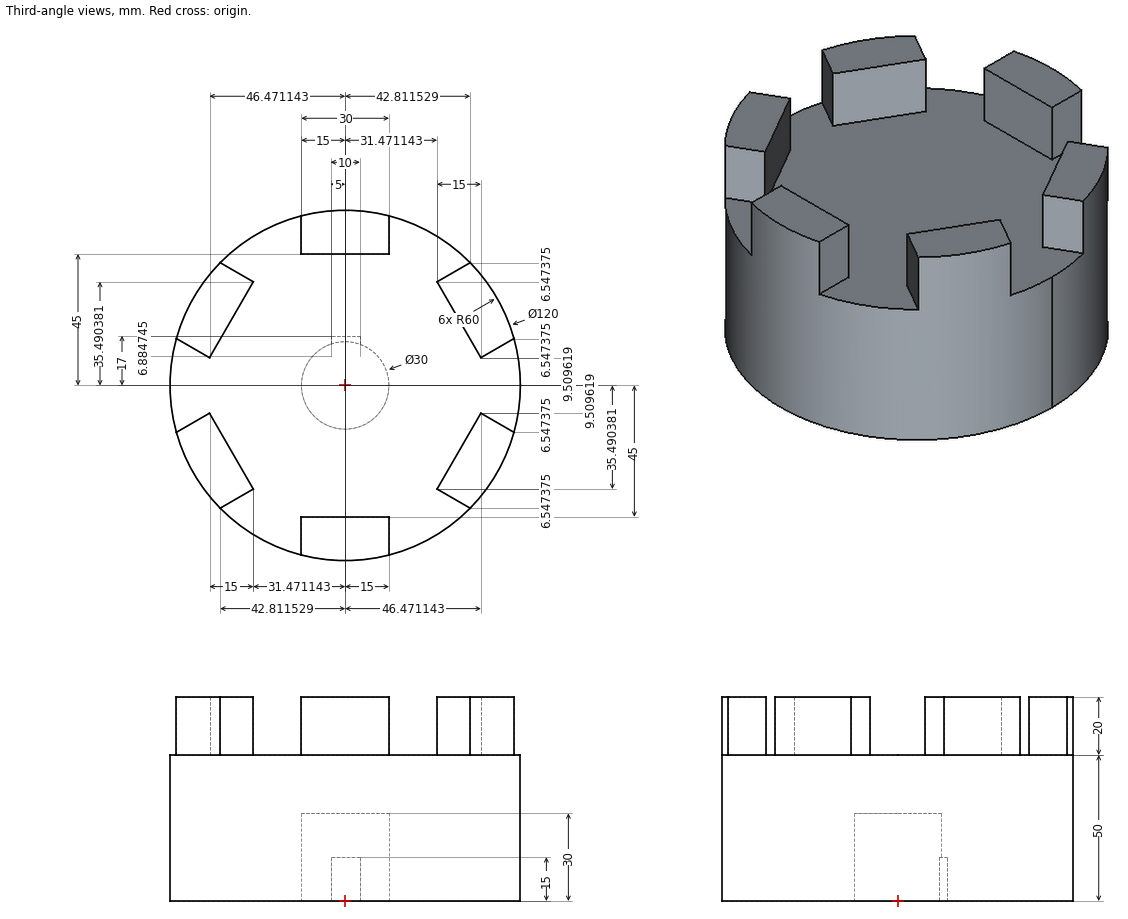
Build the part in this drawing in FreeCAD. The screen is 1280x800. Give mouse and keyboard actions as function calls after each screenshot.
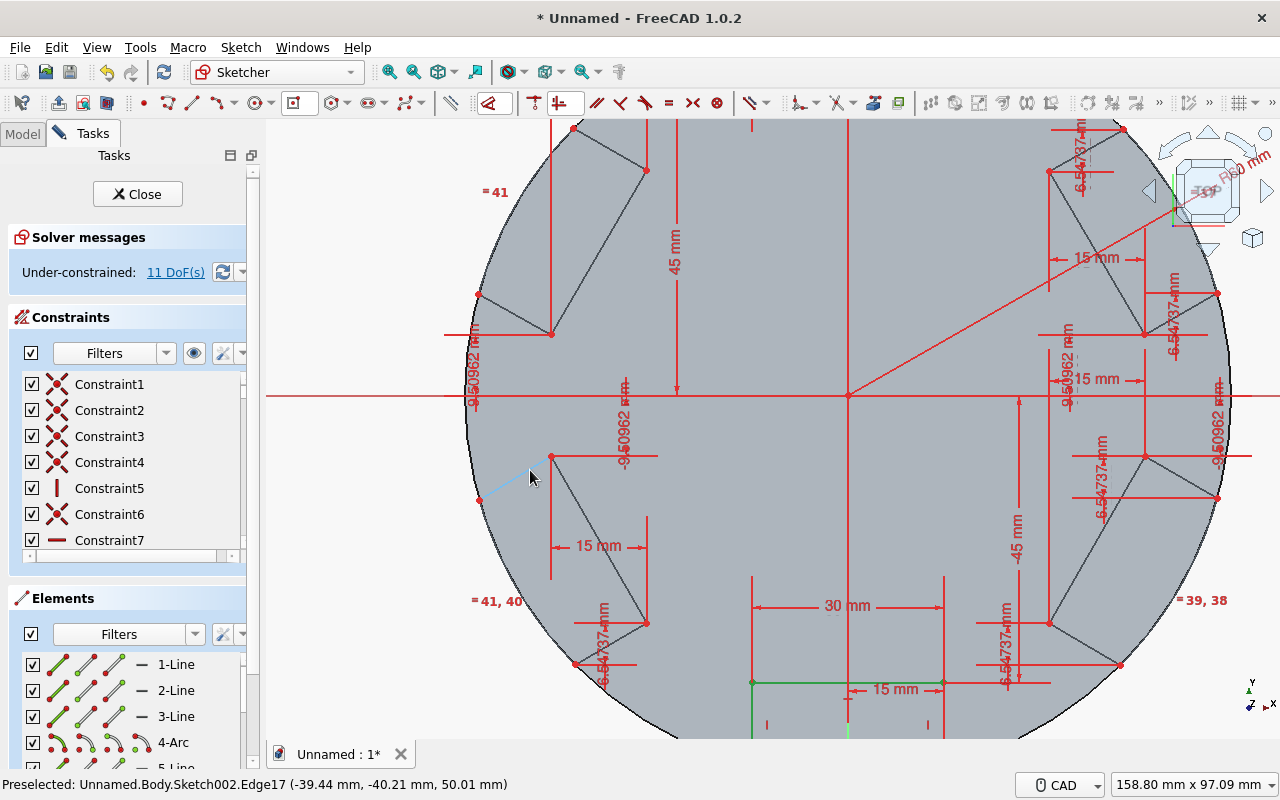
click(530, 470)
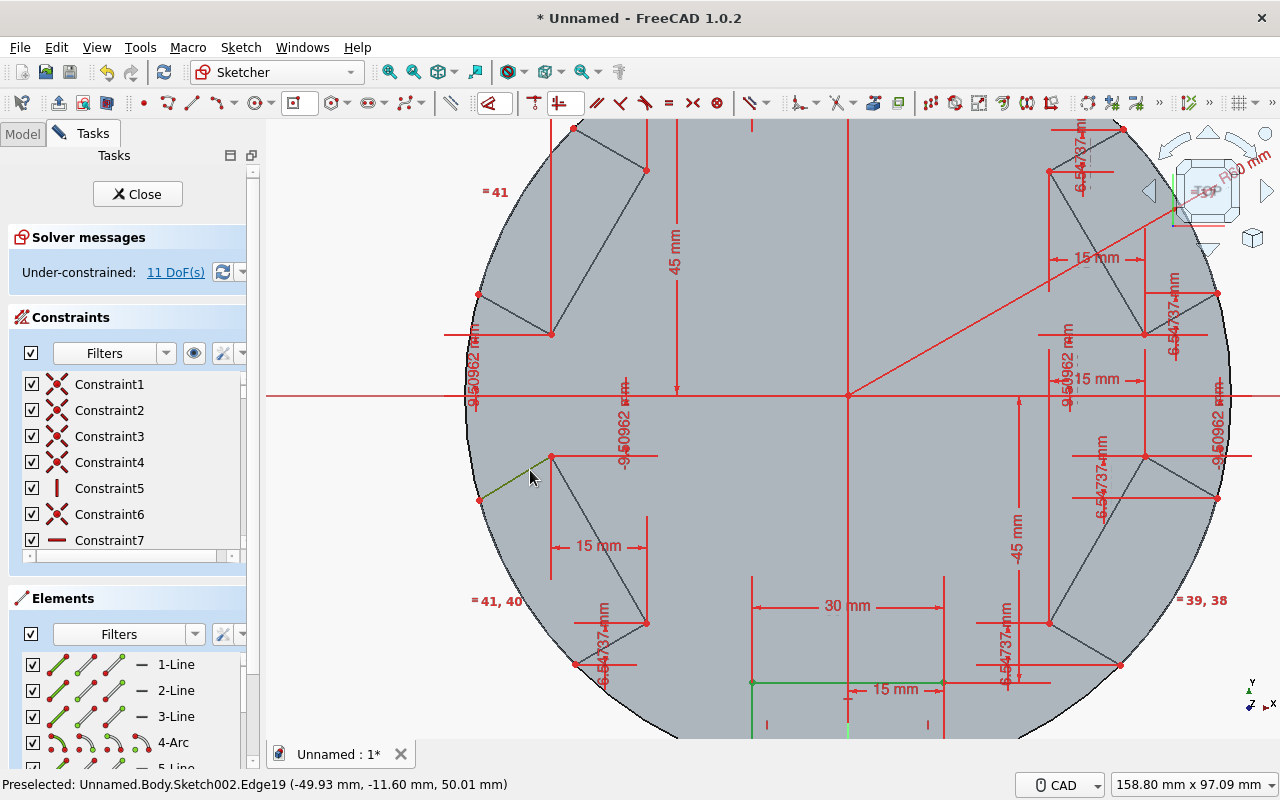
key(i)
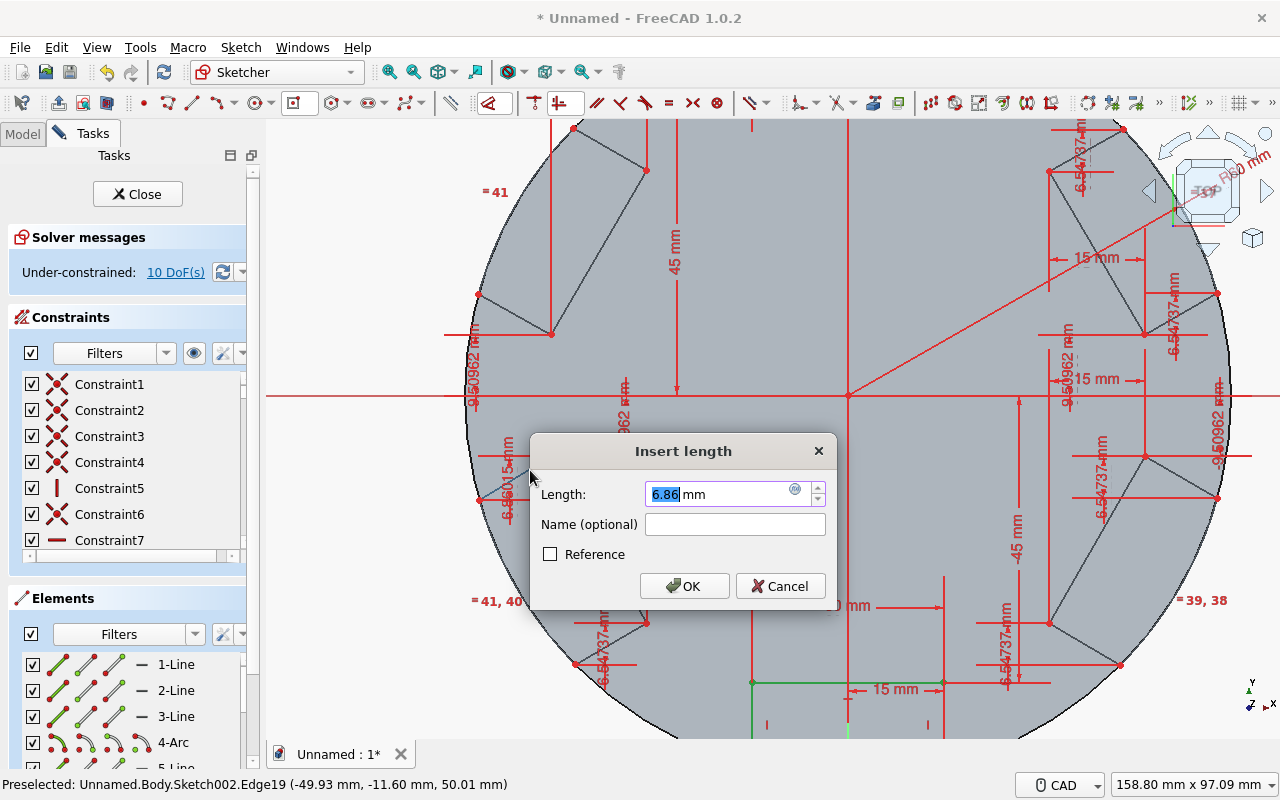
text(6.547375)
key(Return)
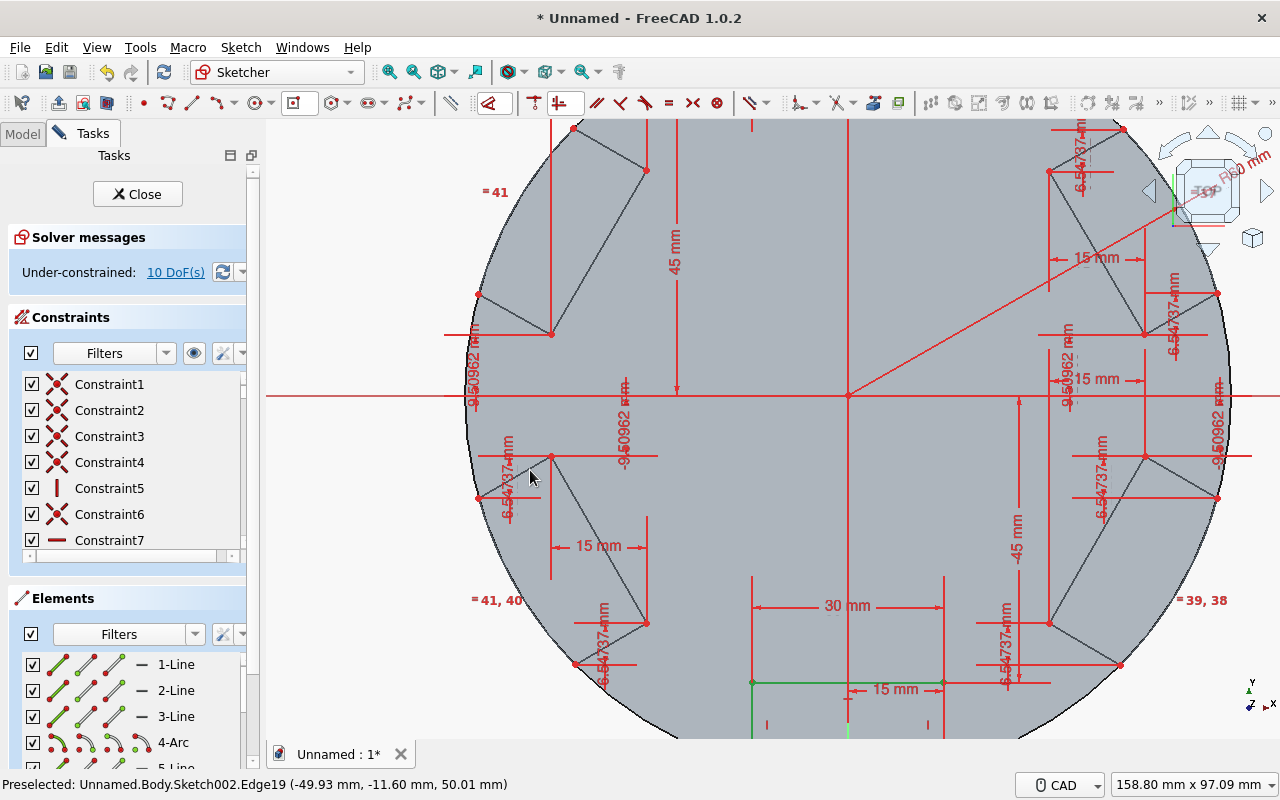
click(500, 306)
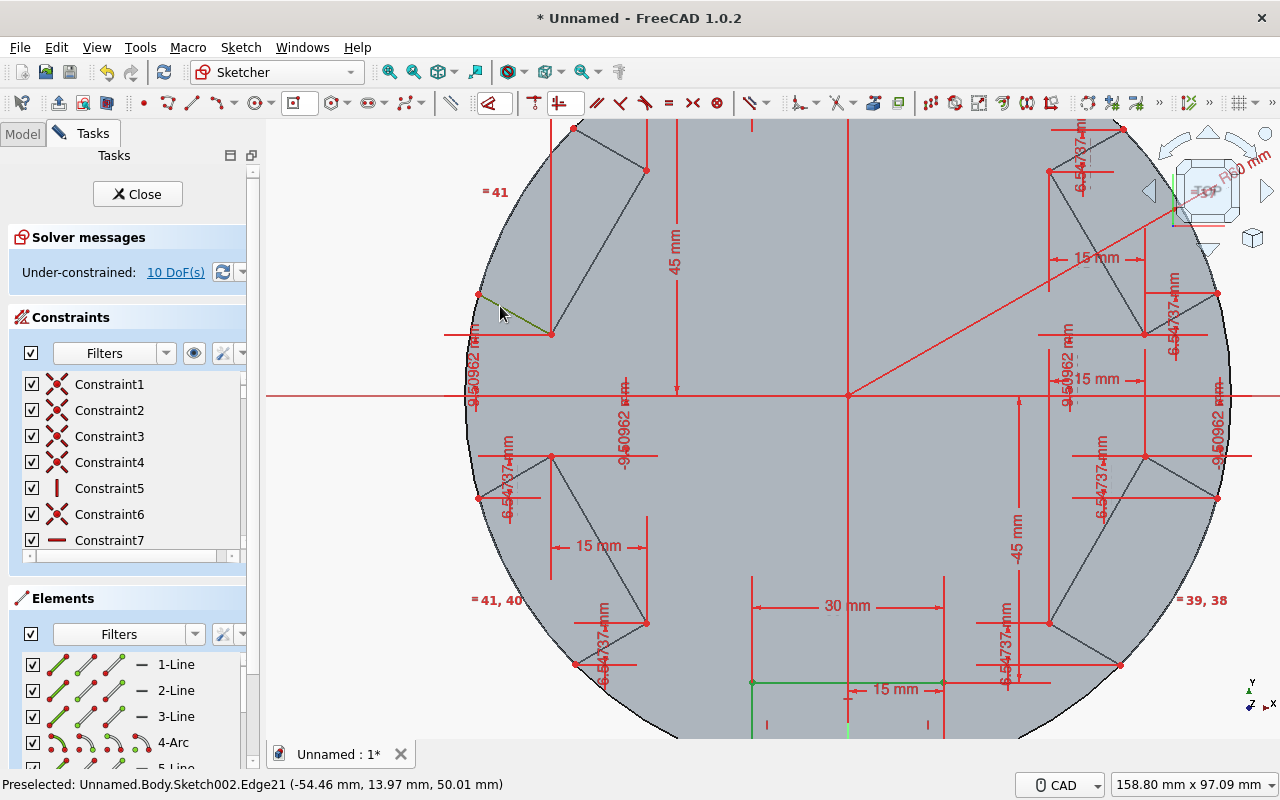
key(i)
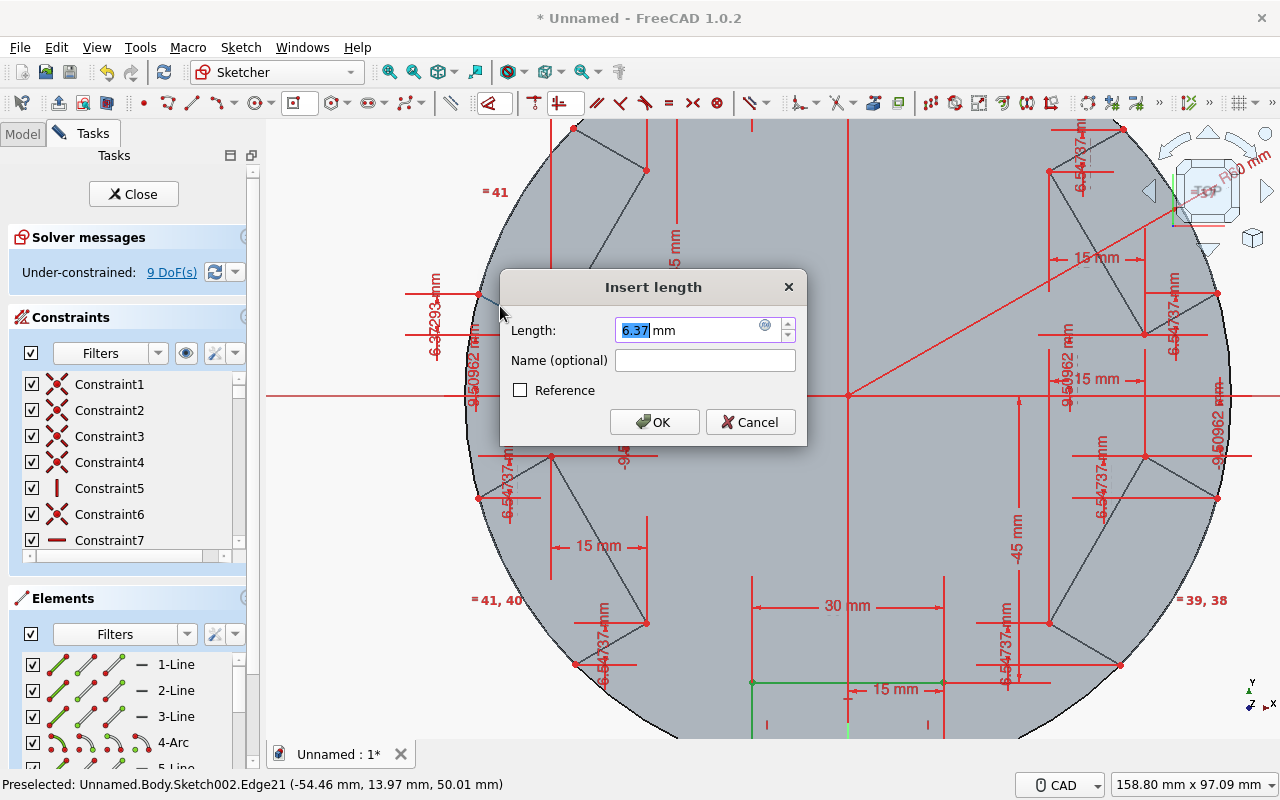
text(6.547375)
key(Return)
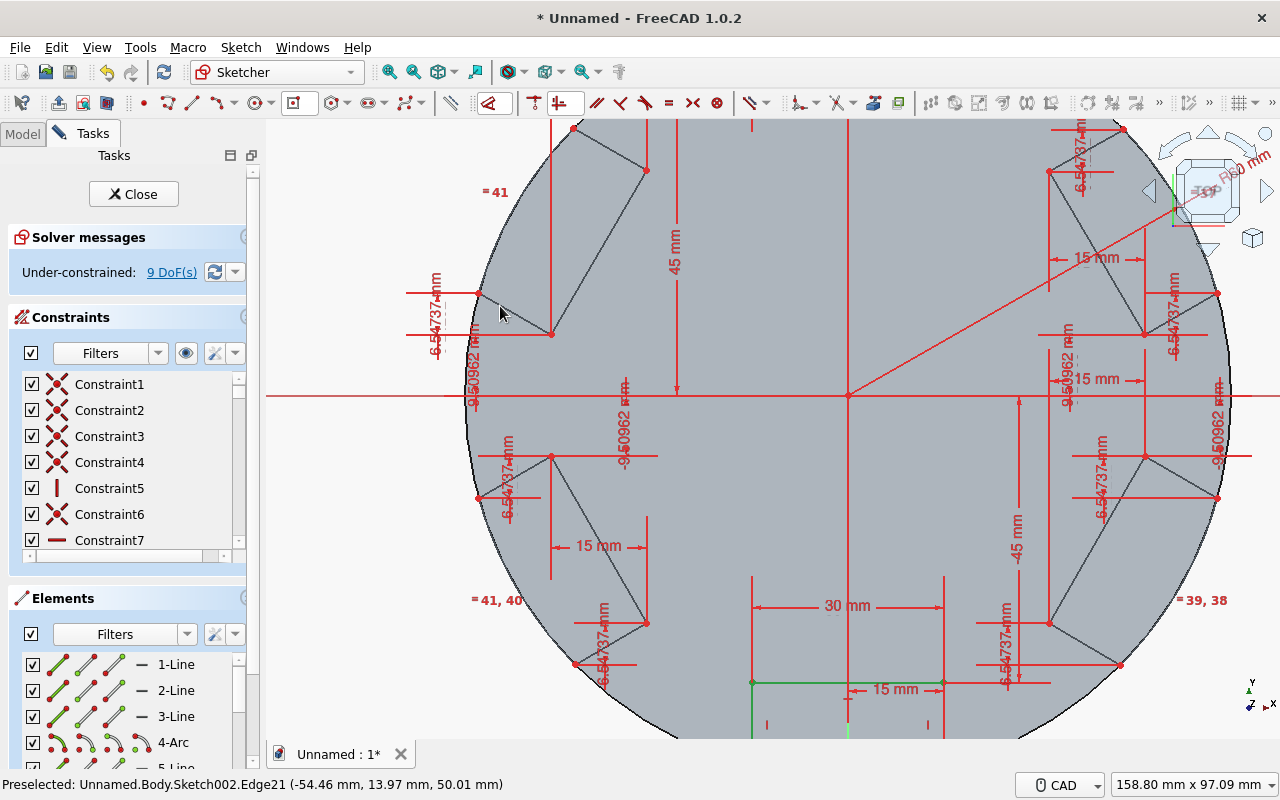
click(625, 158)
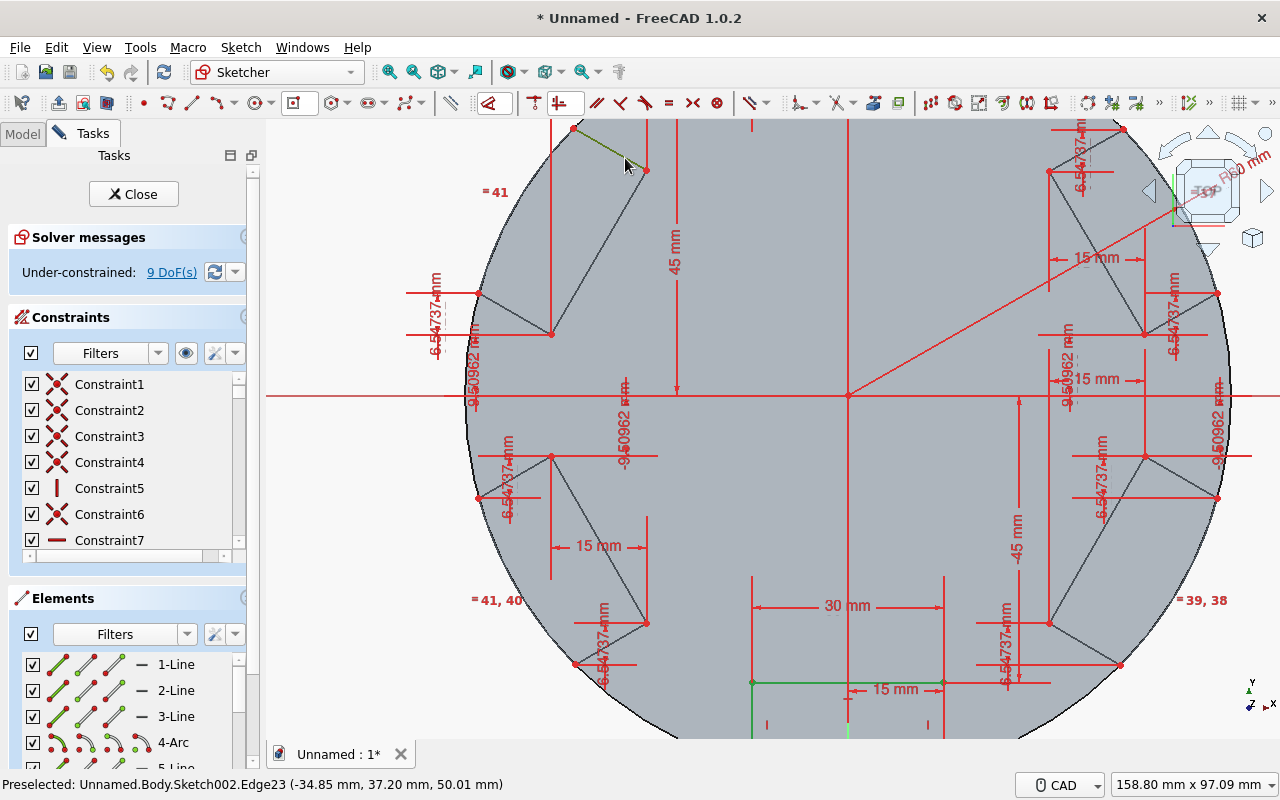
key(i)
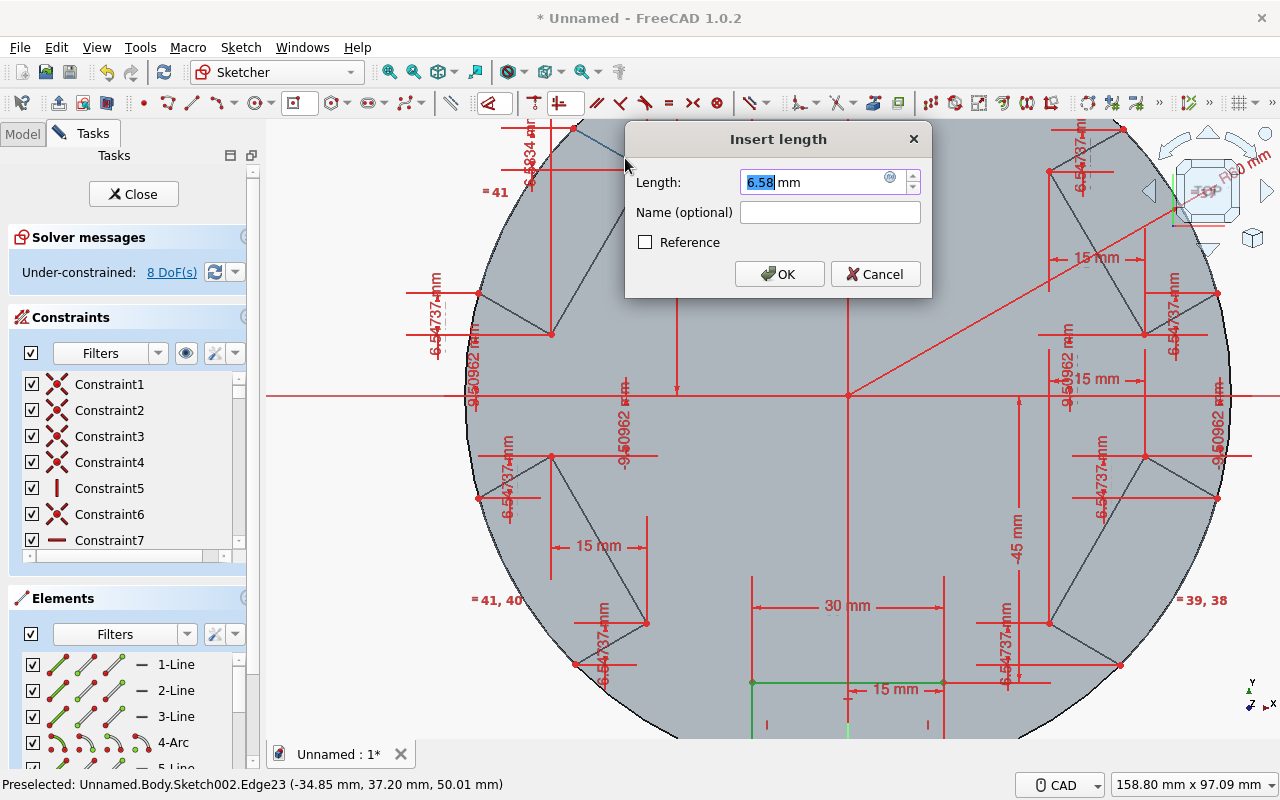
text(6.547375)
key(Return)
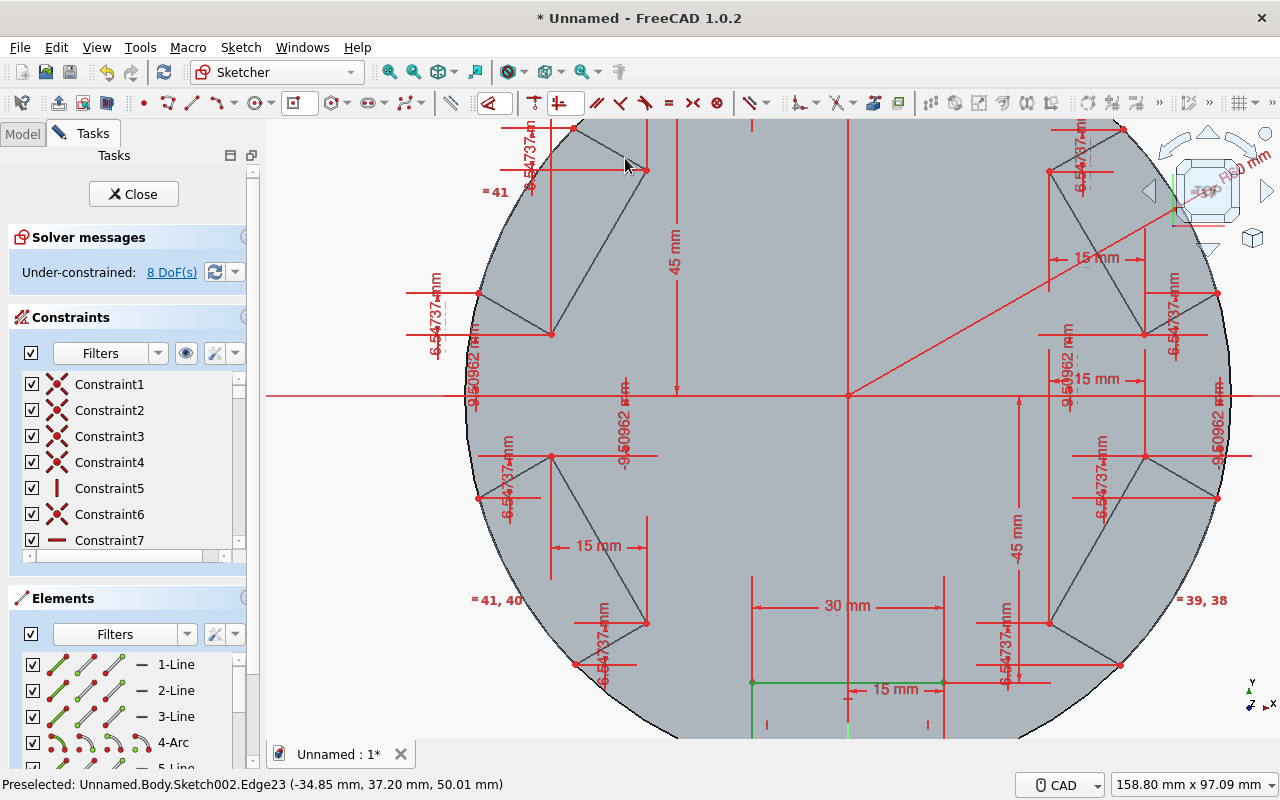
scroll(530, 470, down, 3)